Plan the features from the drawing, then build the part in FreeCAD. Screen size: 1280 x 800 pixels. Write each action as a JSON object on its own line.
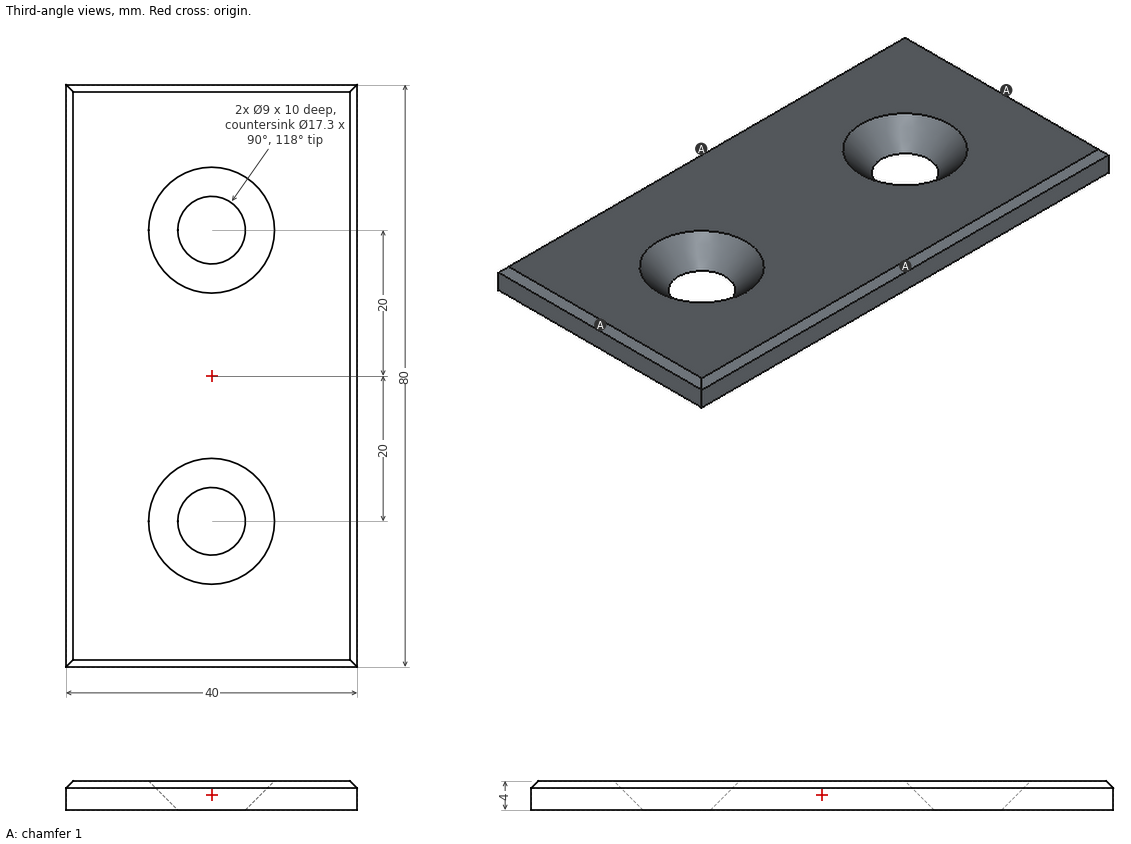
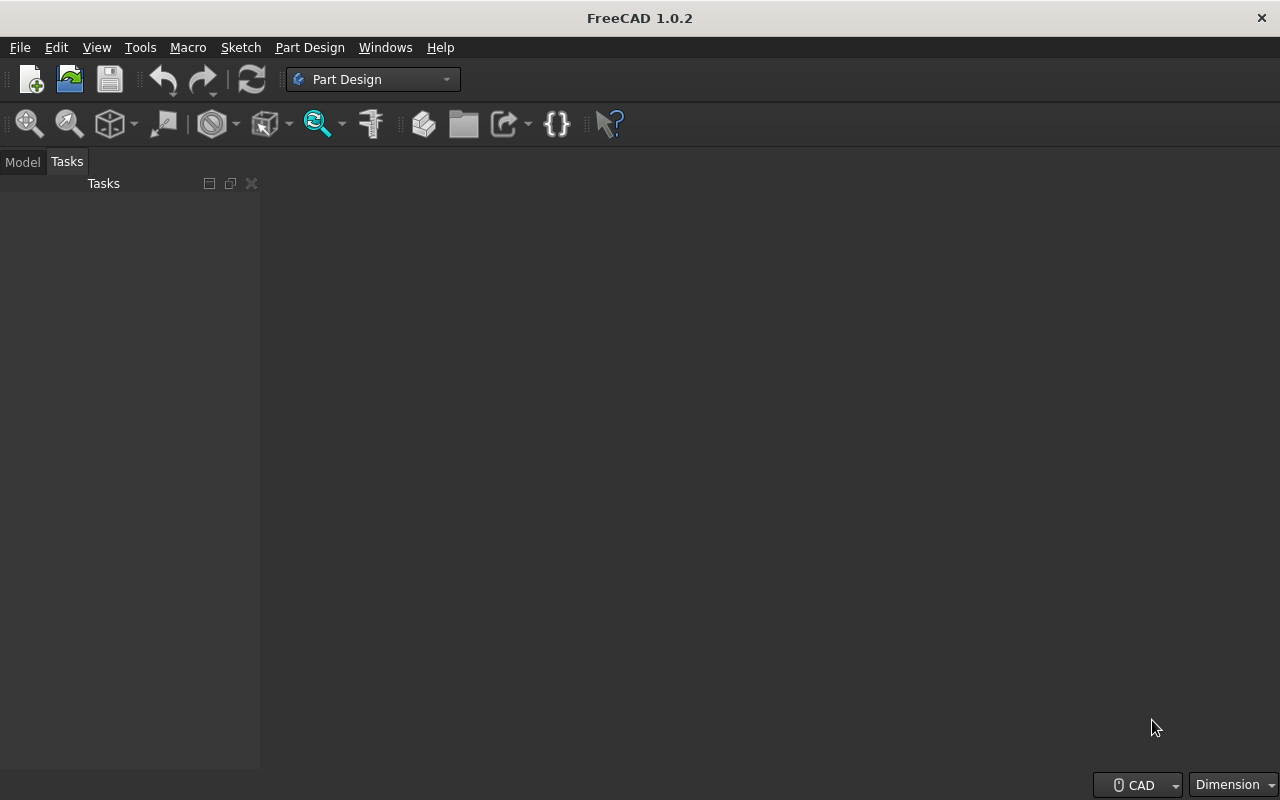
{"action": "key", "text": "ctrl+n"}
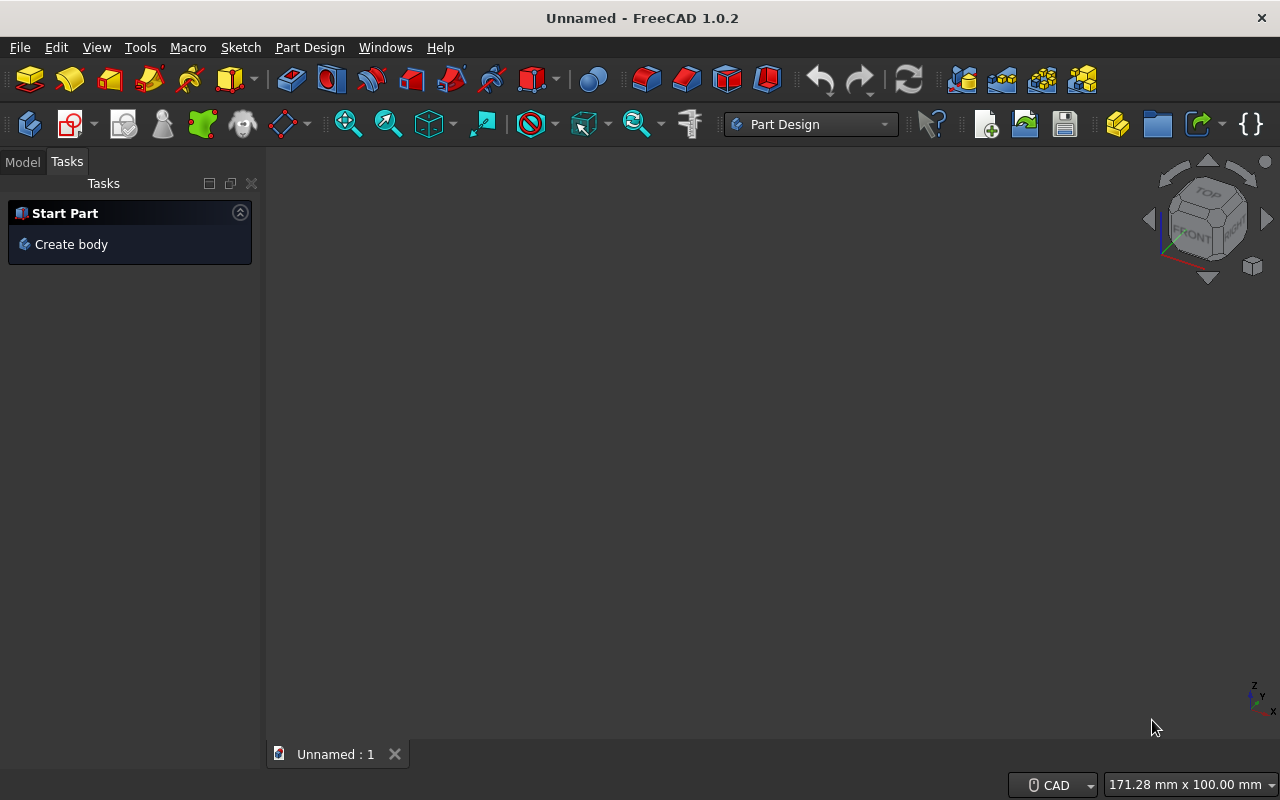
{"action": "left_click", "coordinate": [70, 124]}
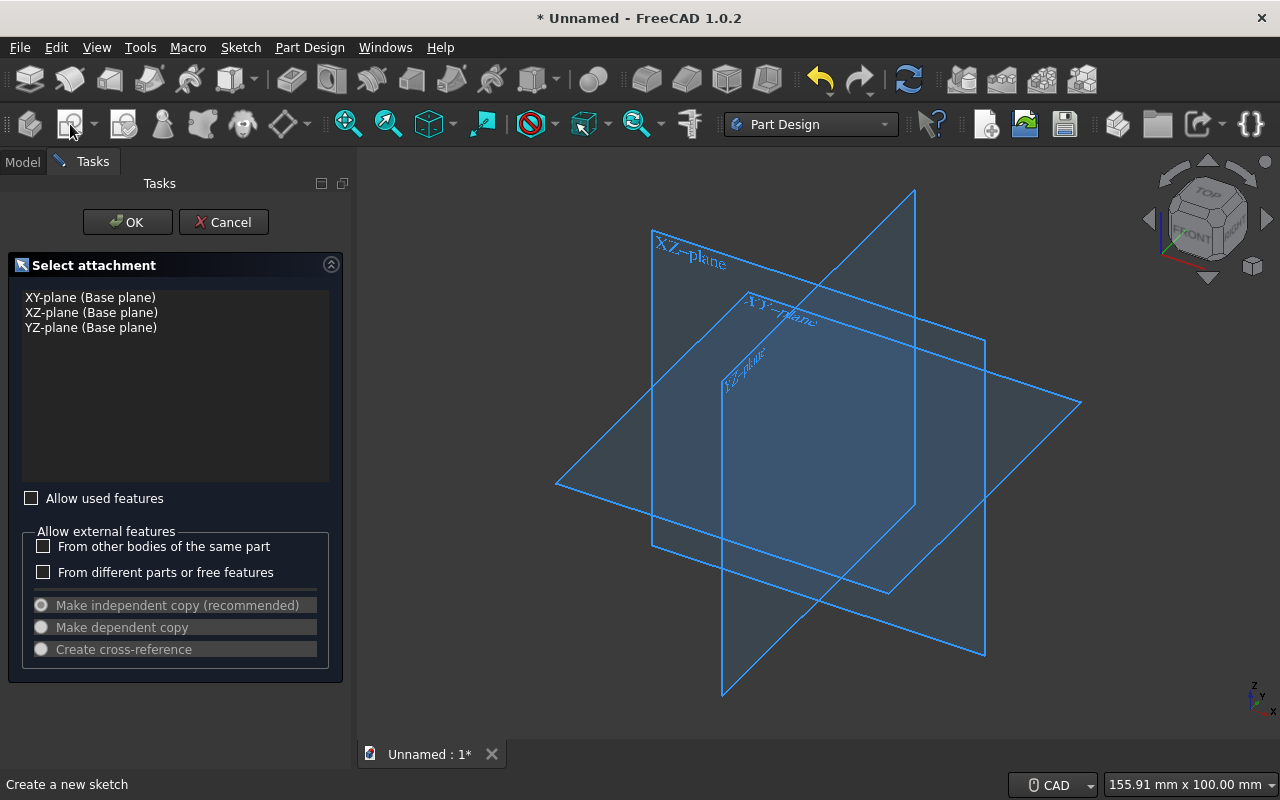
{"action": "left_click", "coordinate": [82, 298]}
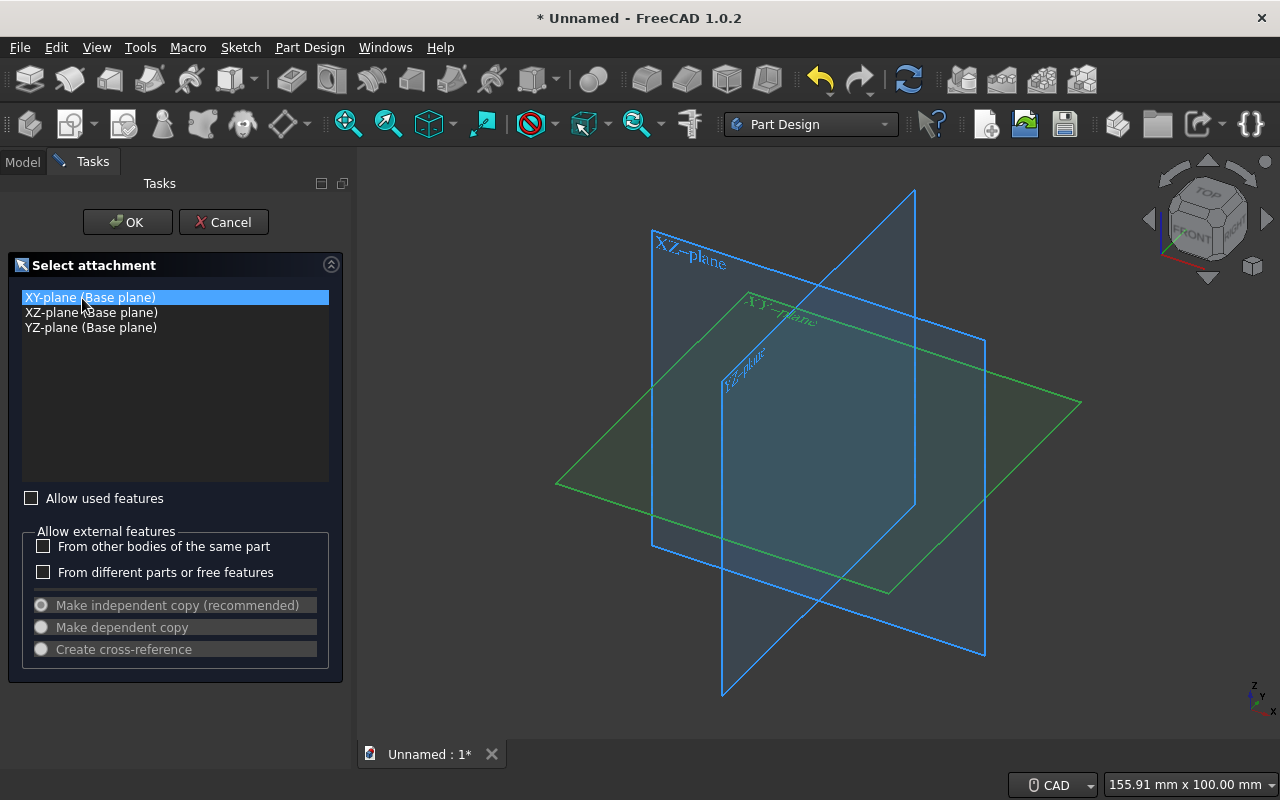
{"action": "left_click", "coordinate": [128, 222]}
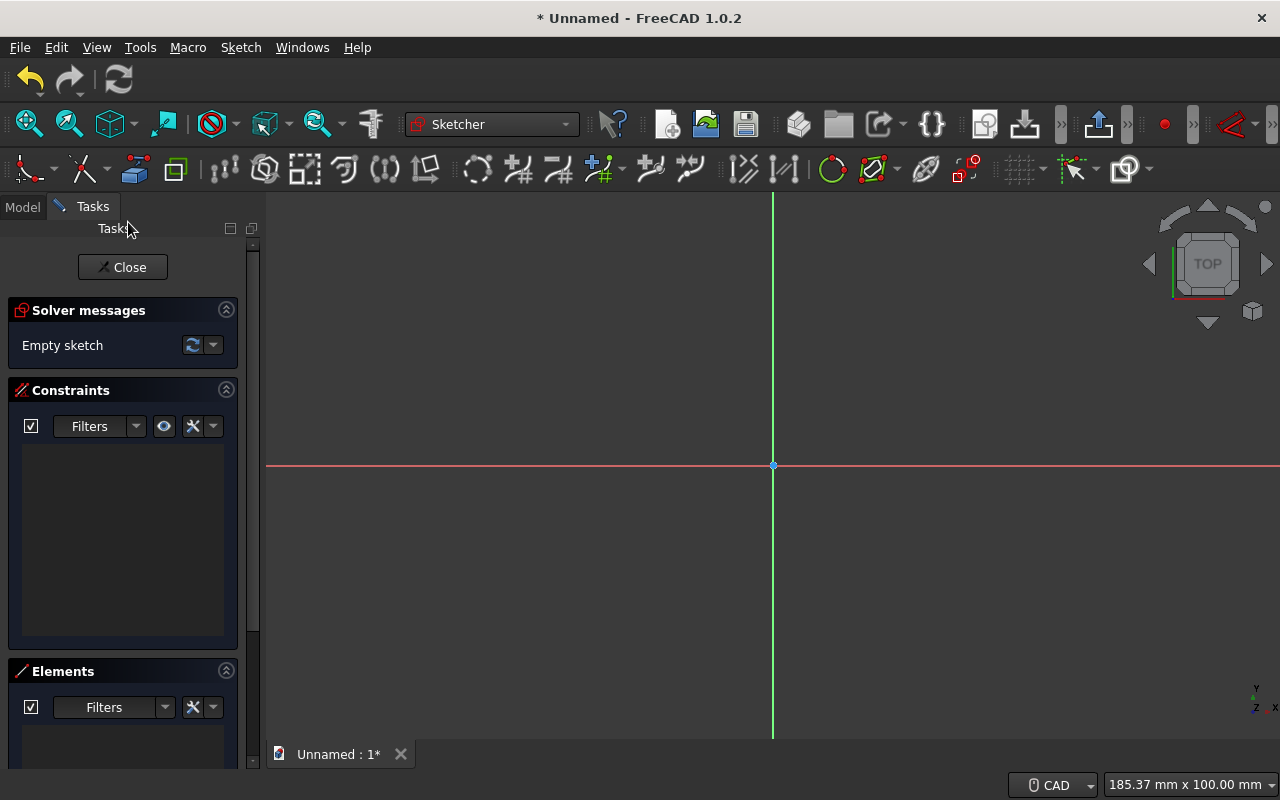
{"action": "key", "text": "g v"}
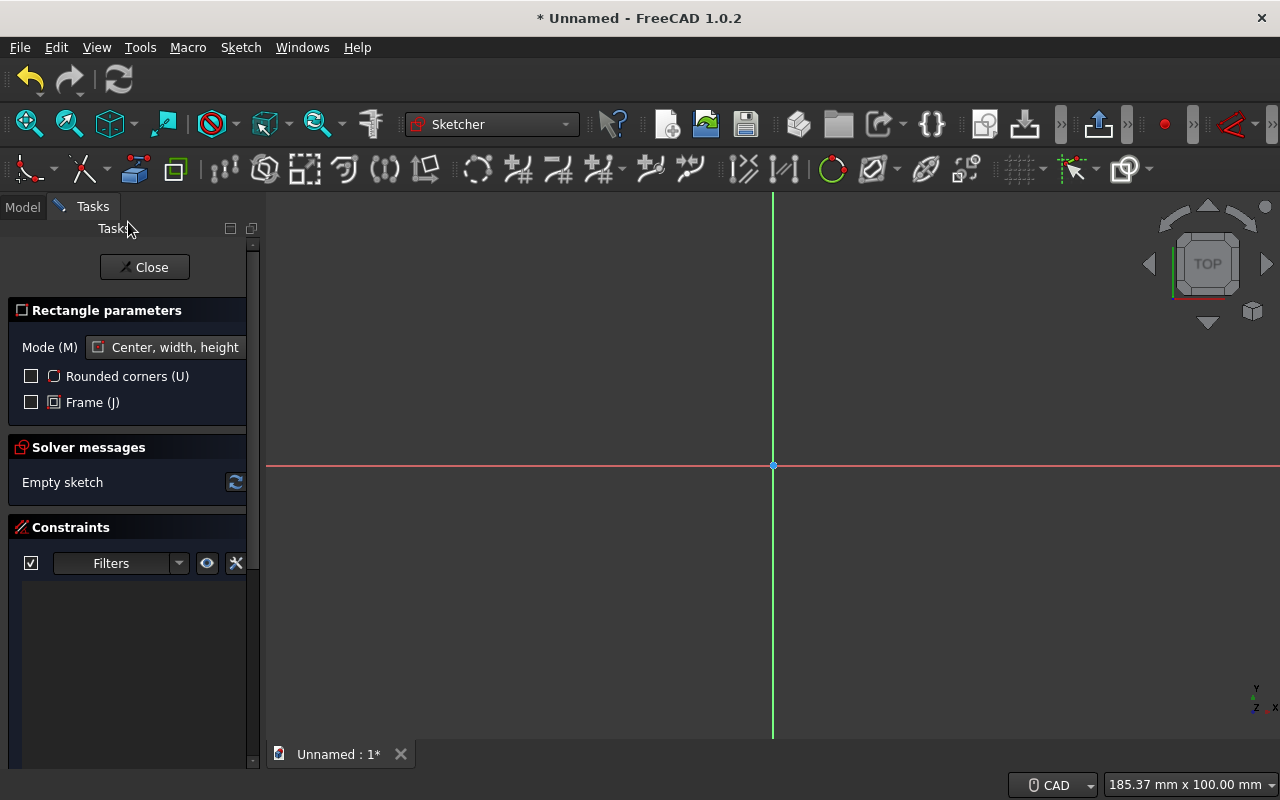
{"action": "left_click", "coordinate": [773, 466]}
{"action": "mouse_move", "coordinate": [882, 247]}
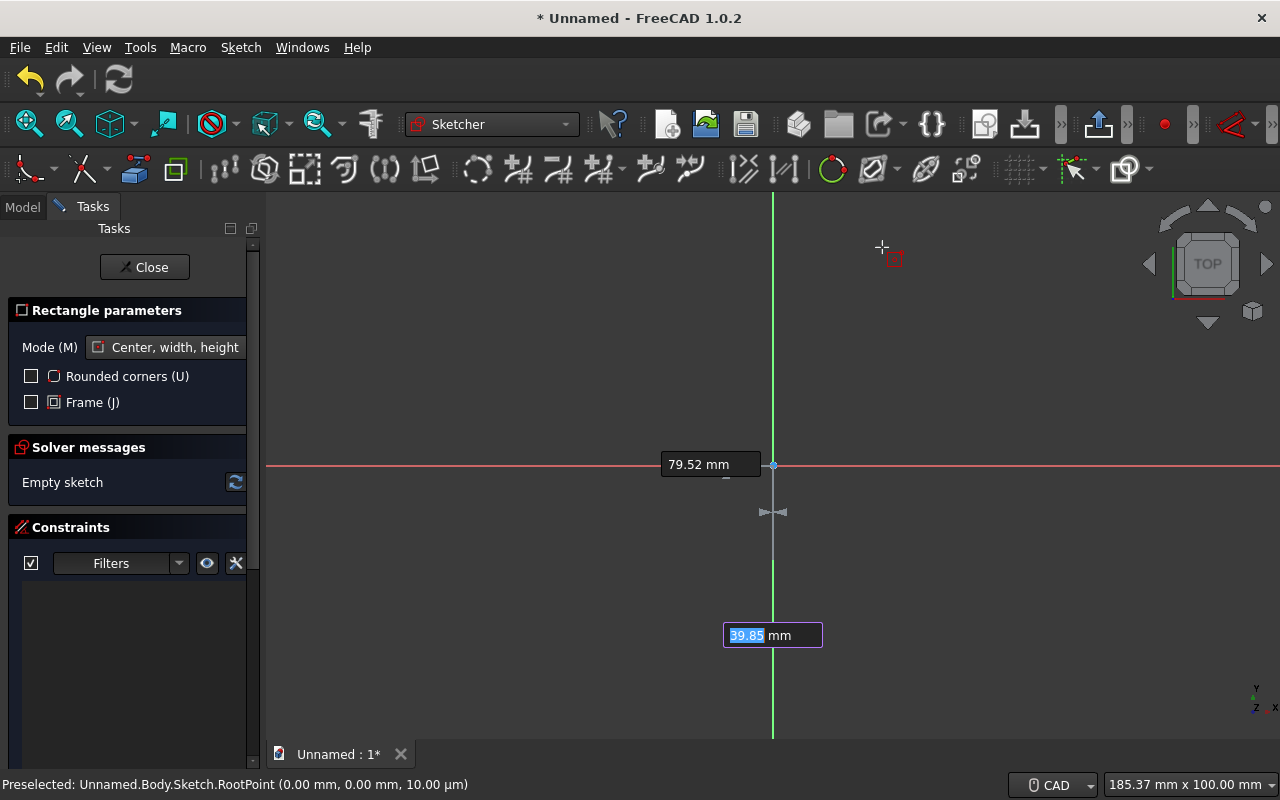
{"action": "type", "text": "40"}
{"action": "key", "text": "Tab"}
{"action": "type", "text": "80"}
{"action": "key", "text": "Return"}
{"action": "key", "text": "Escape"}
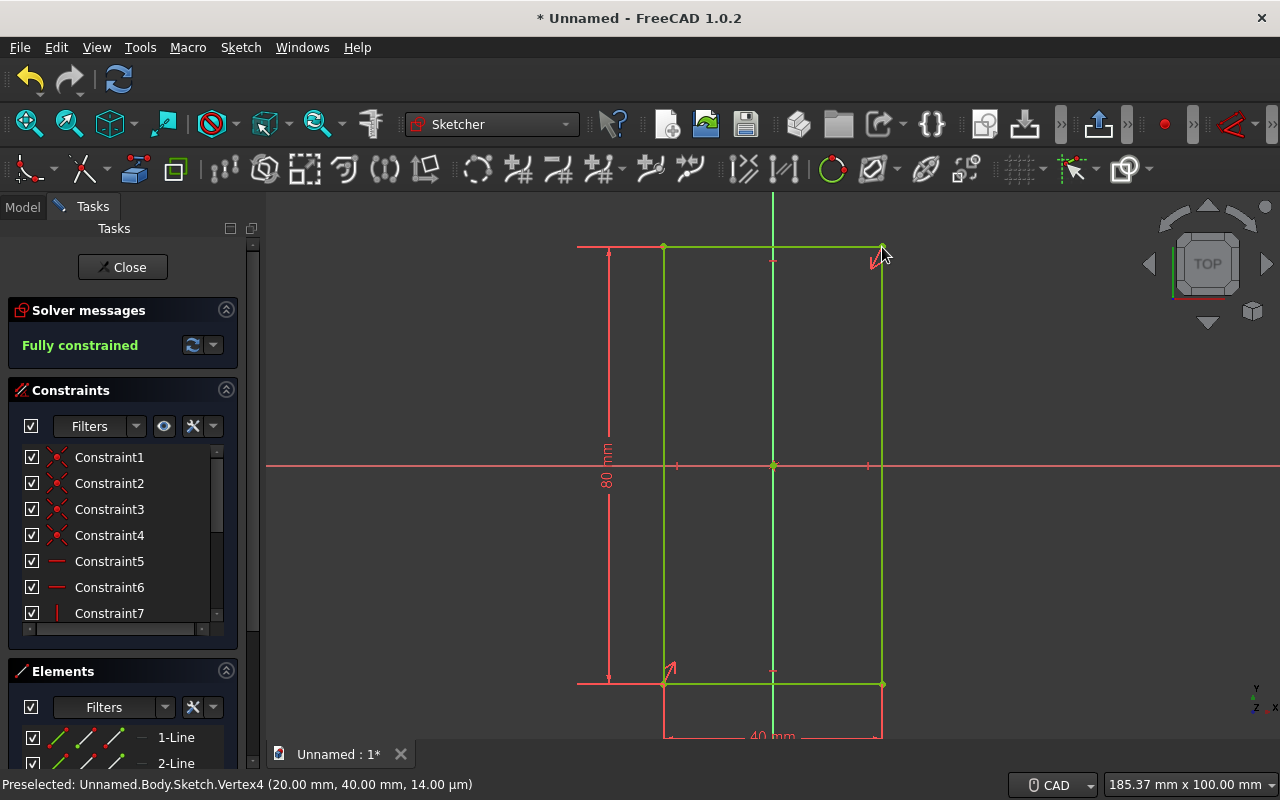
{"action": "left_click", "coordinate": [123, 267]}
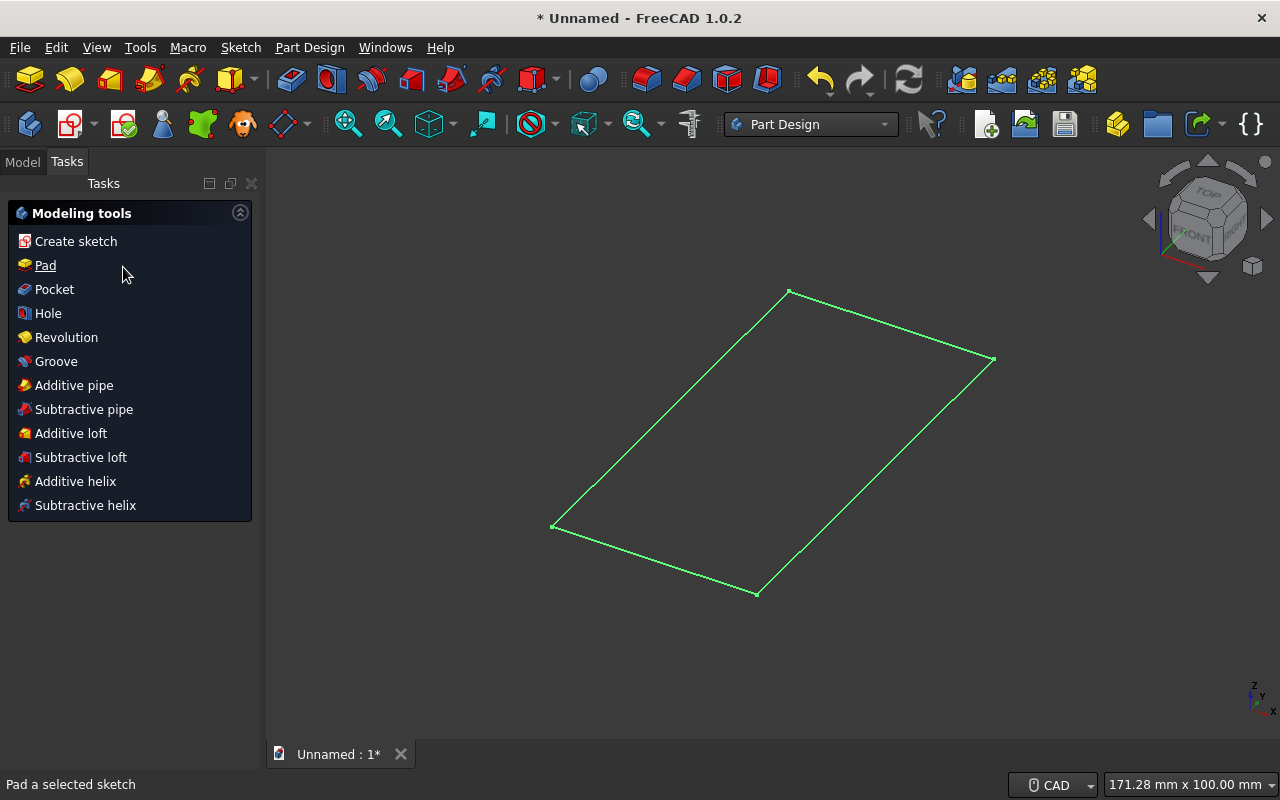
{"action": "left_click", "coordinate": [30, 80]}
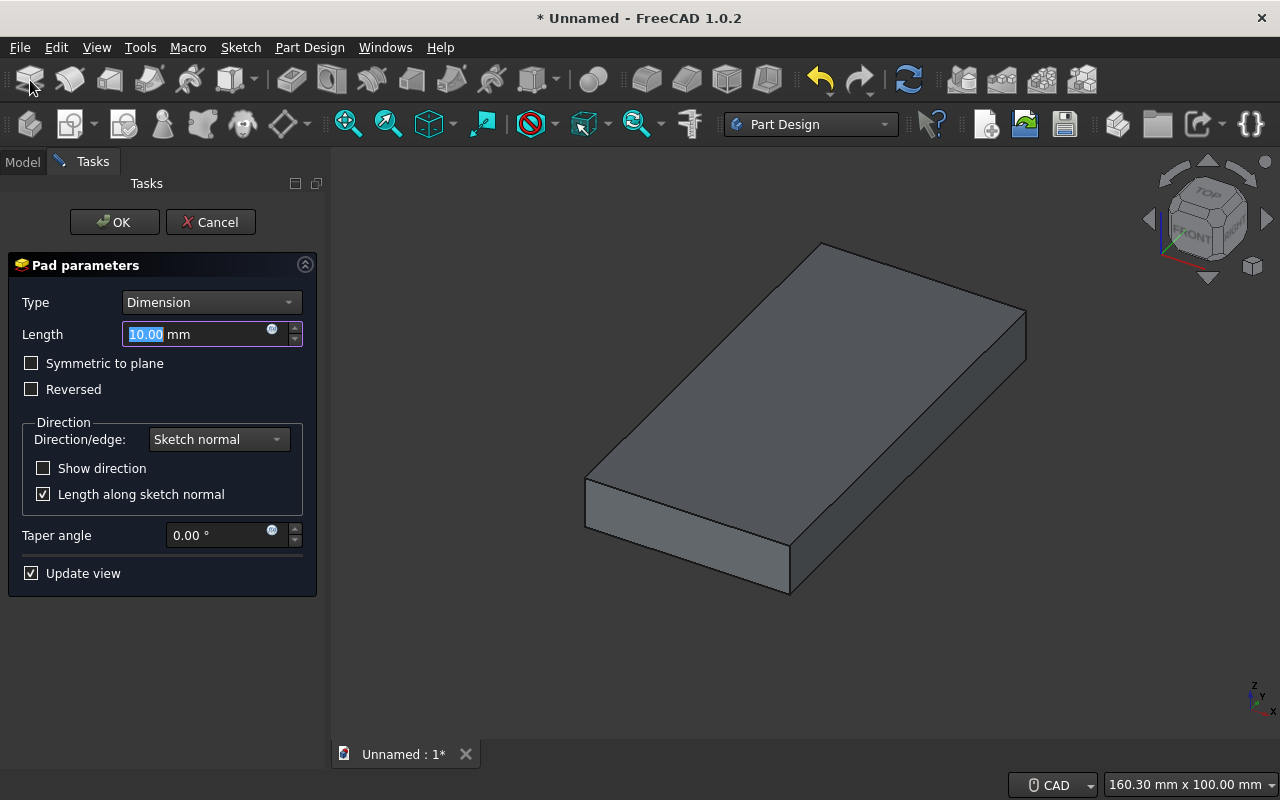
{"action": "type", "text": "4"}
{"action": "key", "text": "Tab"}